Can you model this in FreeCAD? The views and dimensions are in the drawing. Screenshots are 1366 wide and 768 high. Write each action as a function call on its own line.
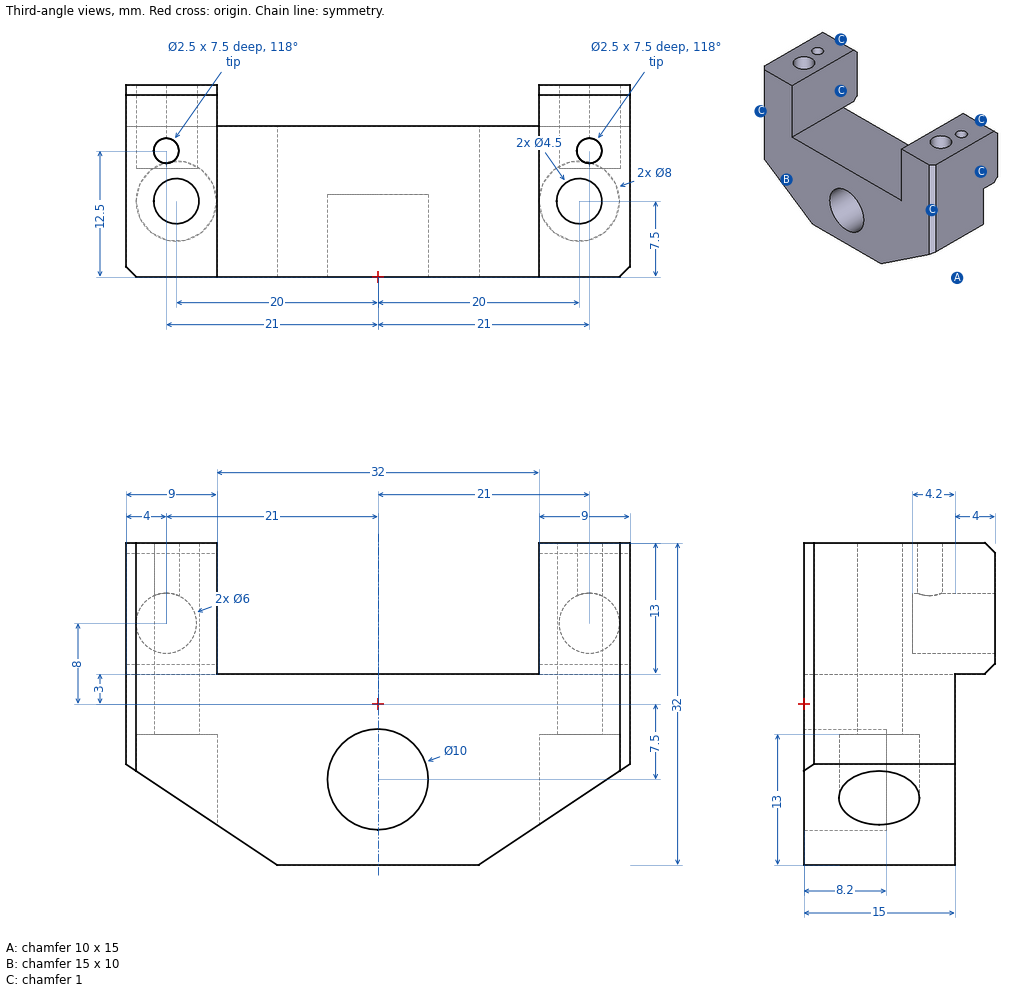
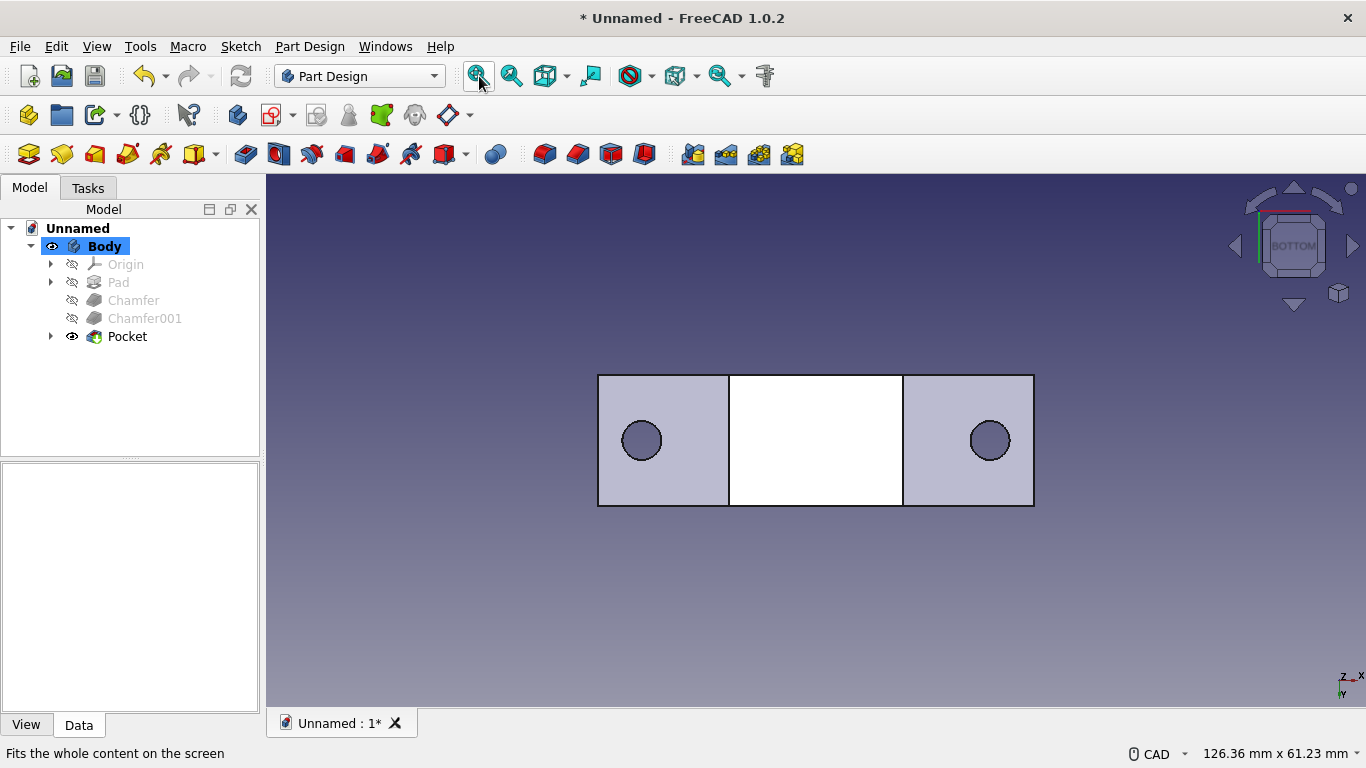
click(816, 439)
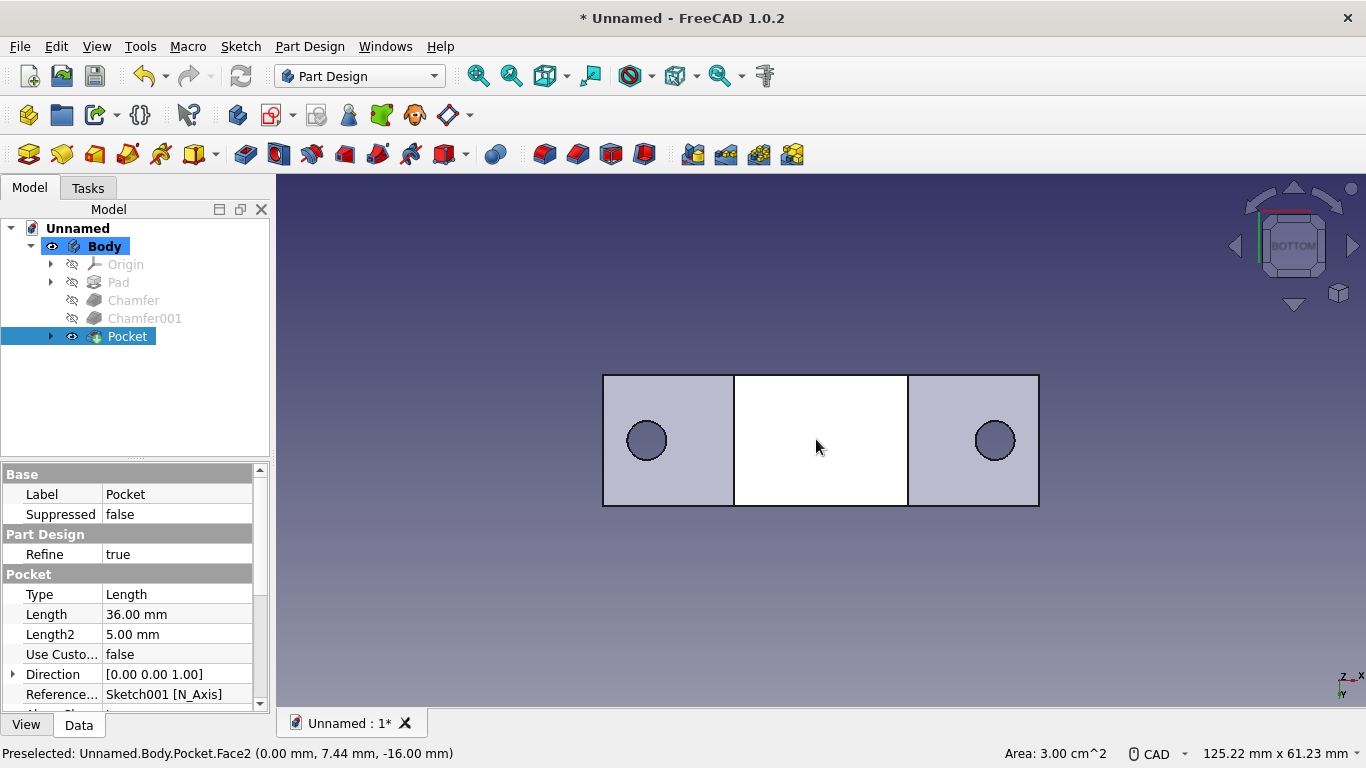
click(270, 116)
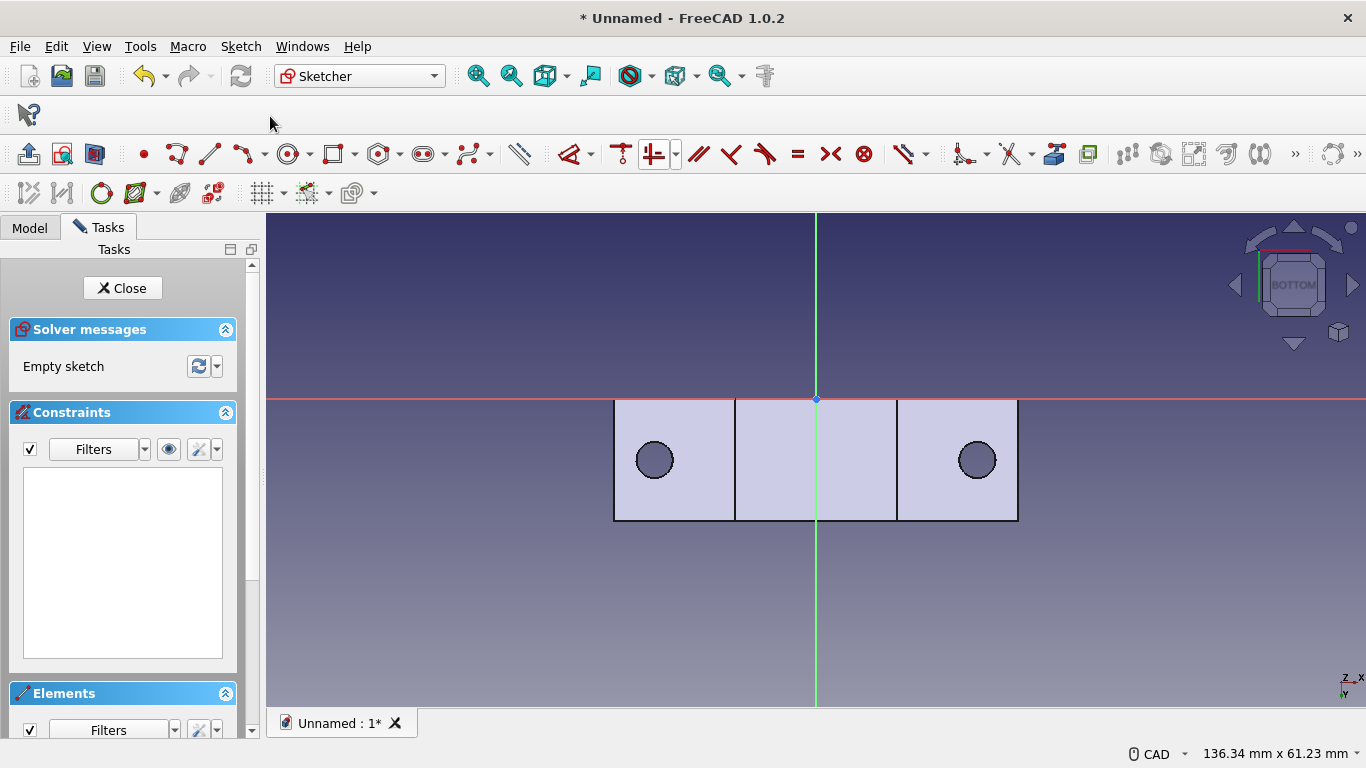
scroll(899, 429, up, 3)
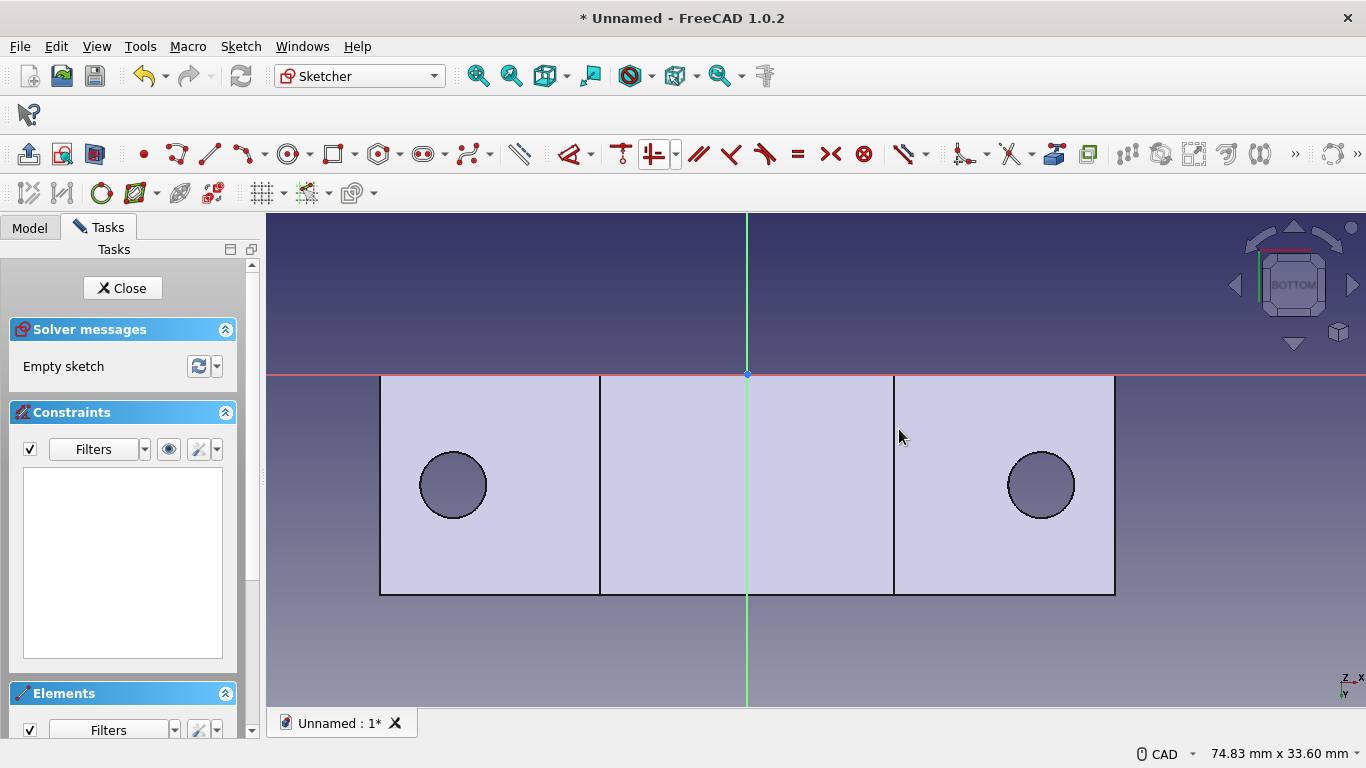
click(288, 154)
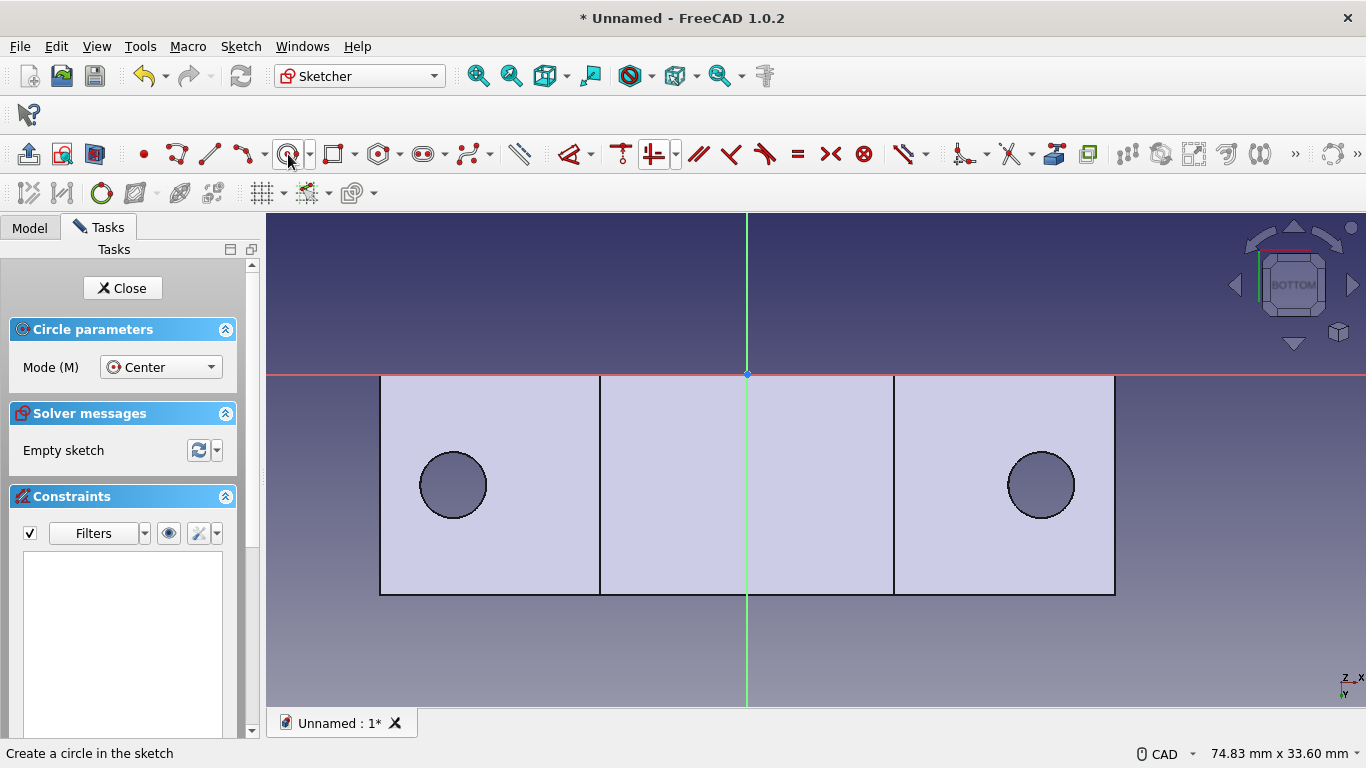
click(1041, 485)
move(1083, 444)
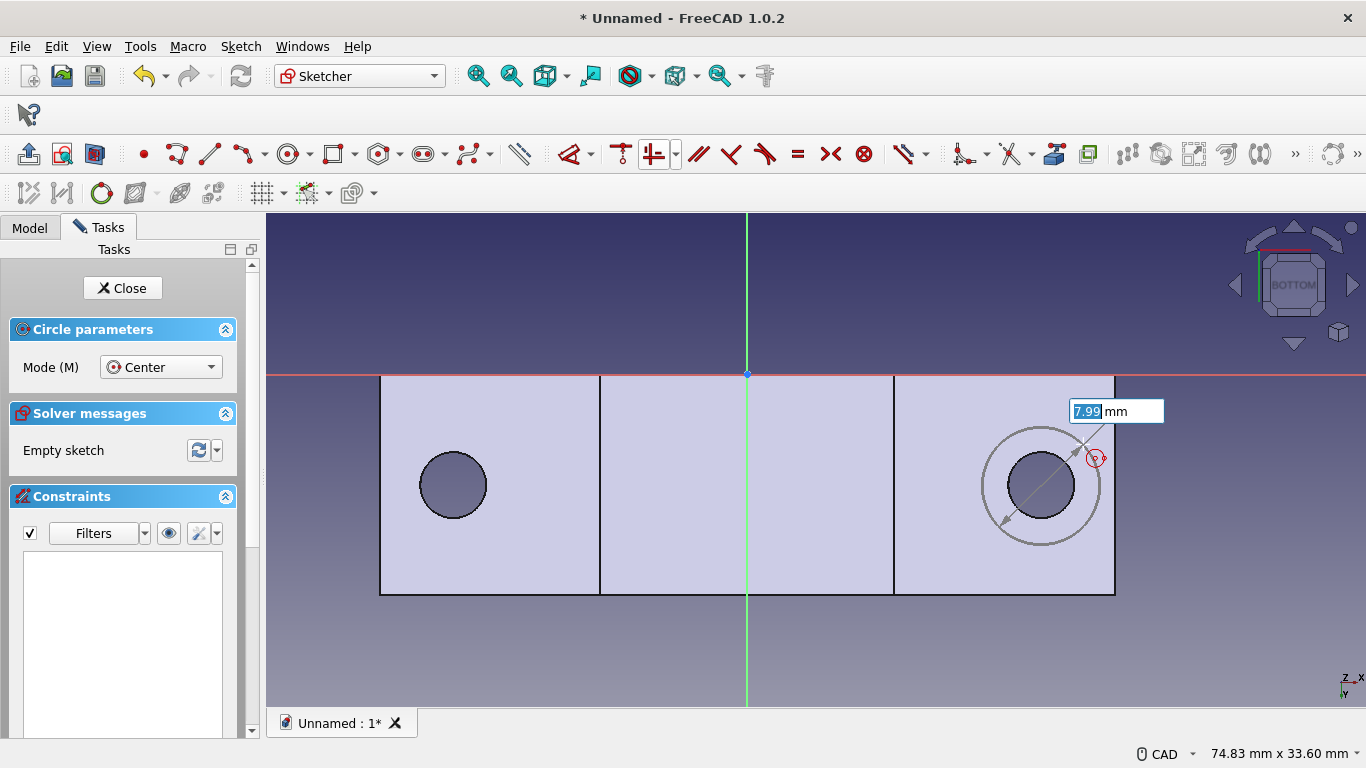
text(8)
key(Return)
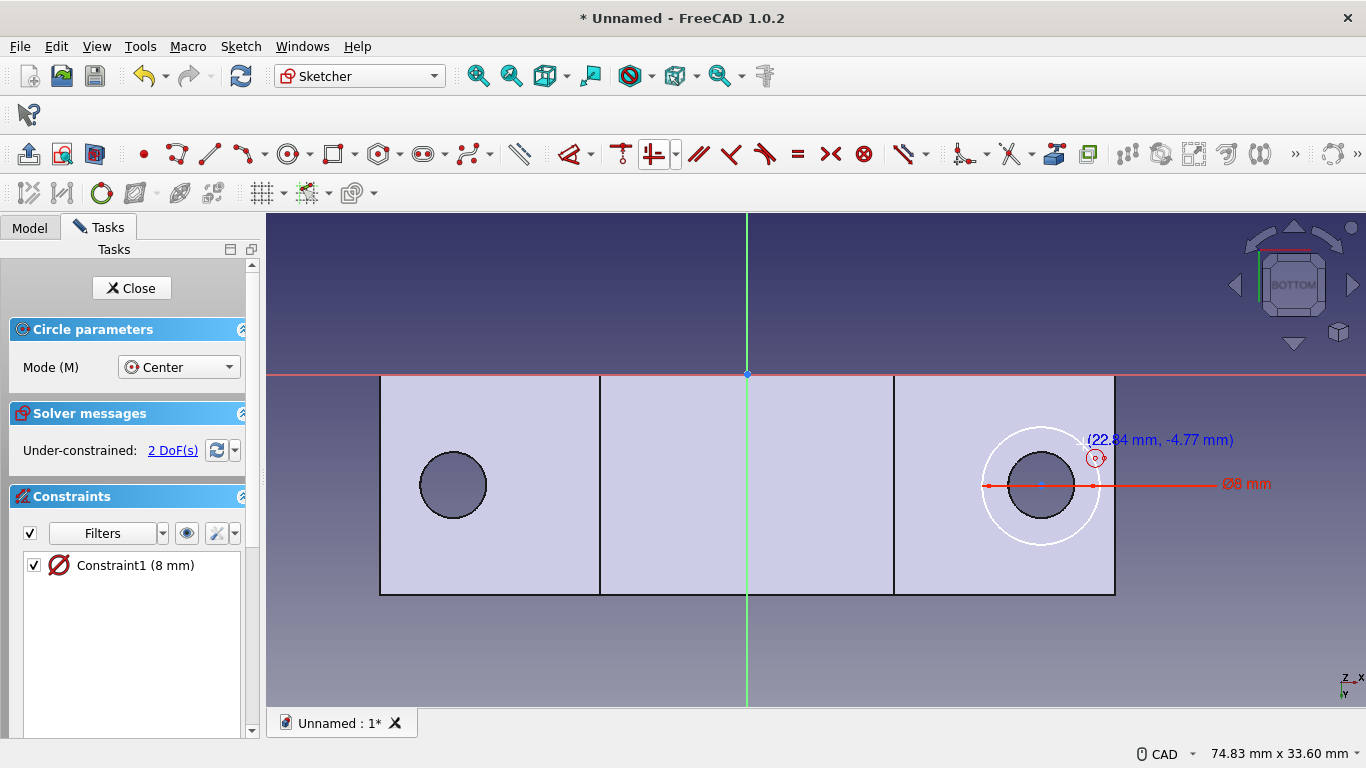
click(453, 485)
move(495, 444)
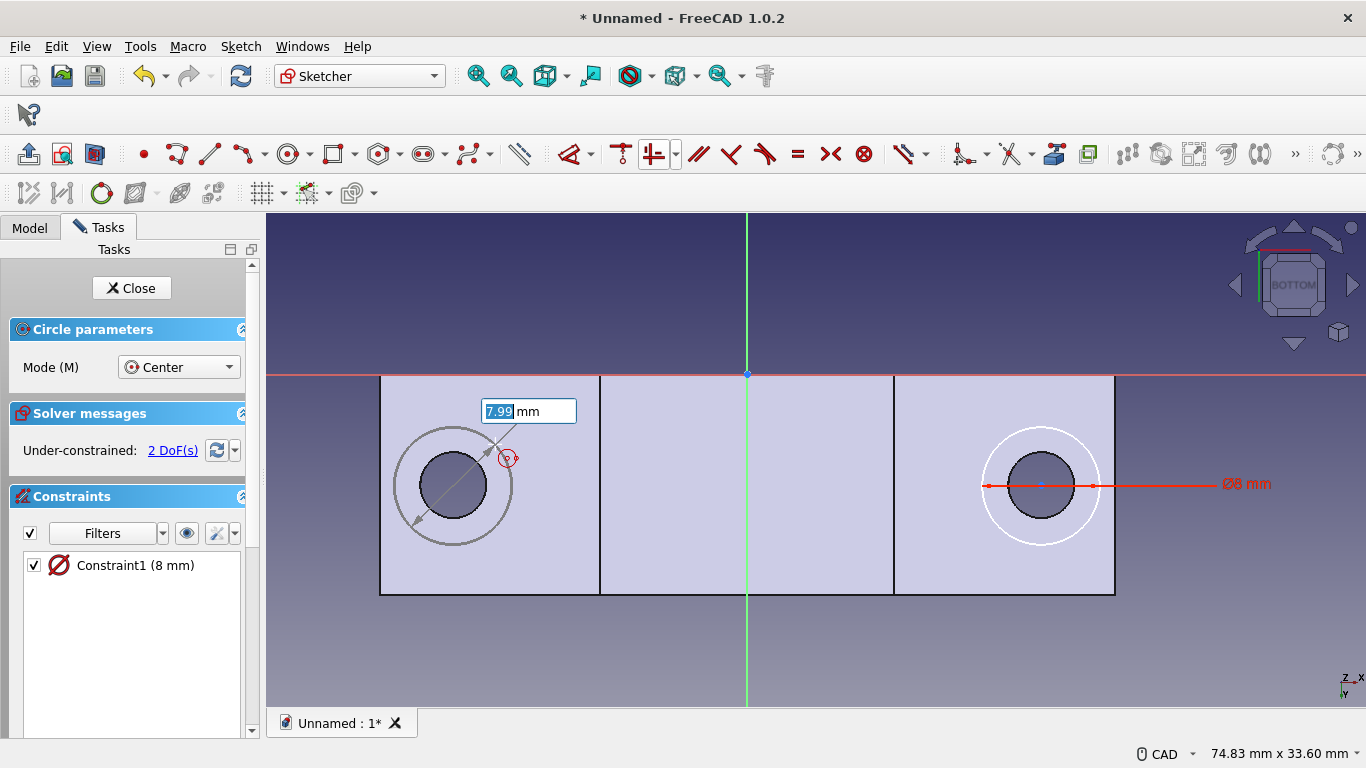
text(8)
key(Return)
key(Escape)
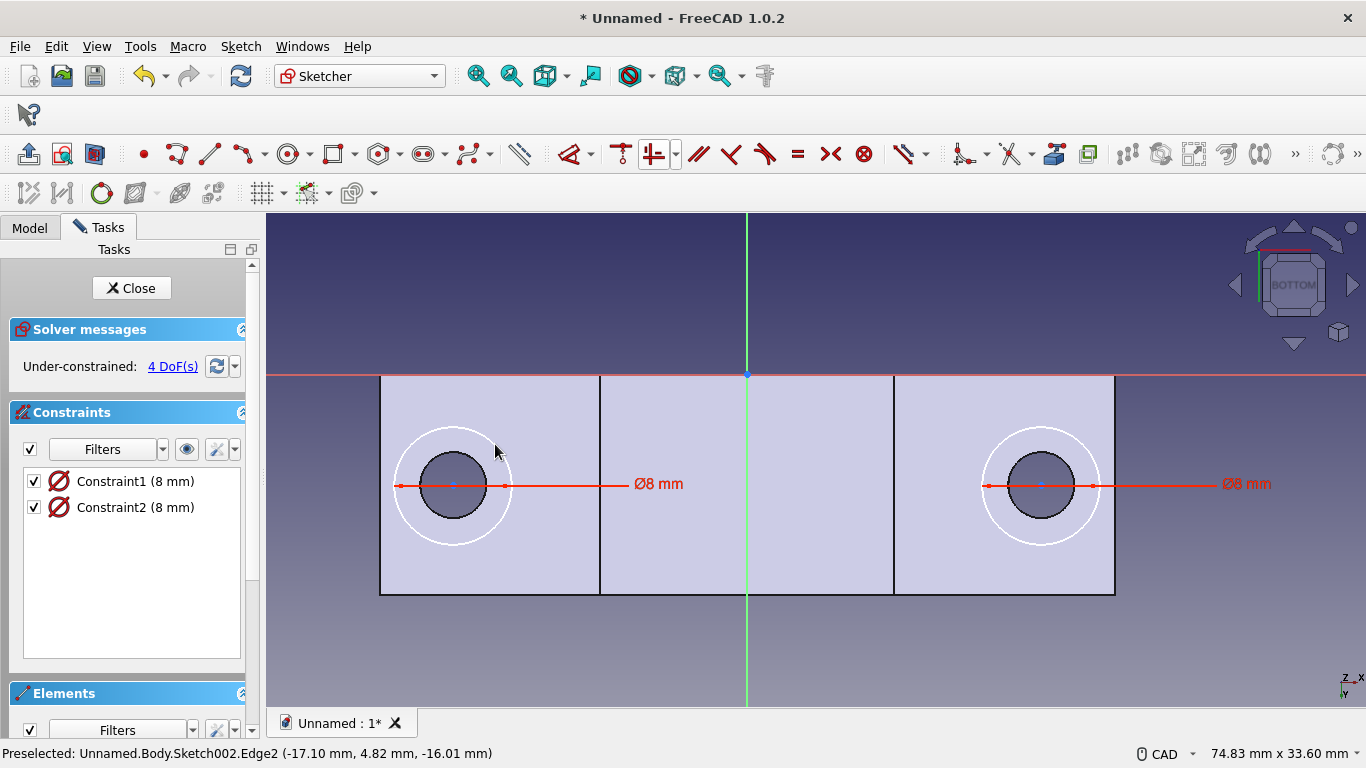
click(1041, 486)